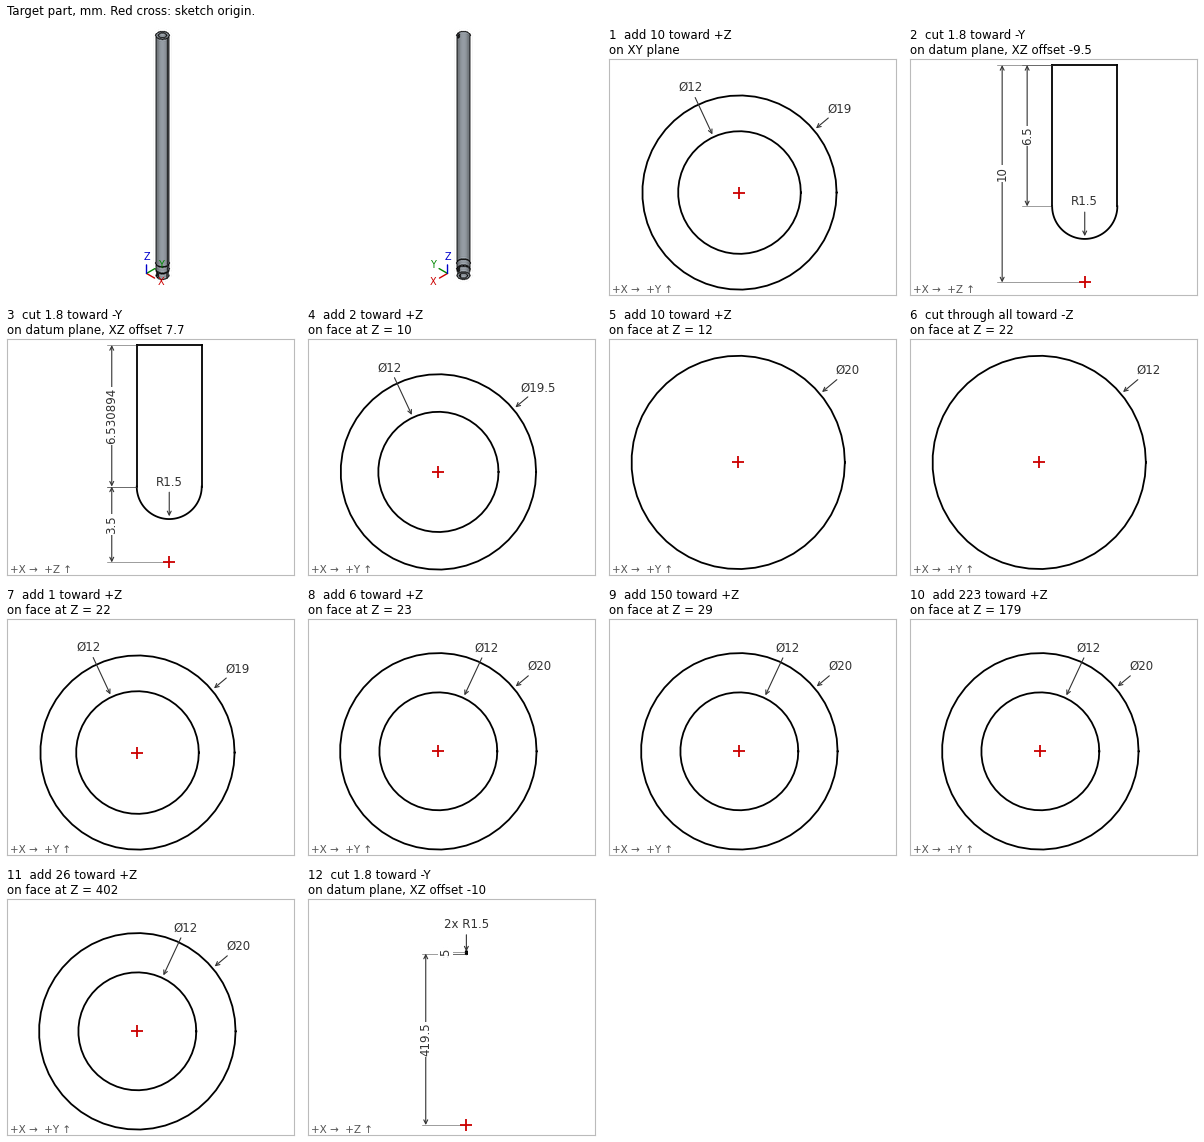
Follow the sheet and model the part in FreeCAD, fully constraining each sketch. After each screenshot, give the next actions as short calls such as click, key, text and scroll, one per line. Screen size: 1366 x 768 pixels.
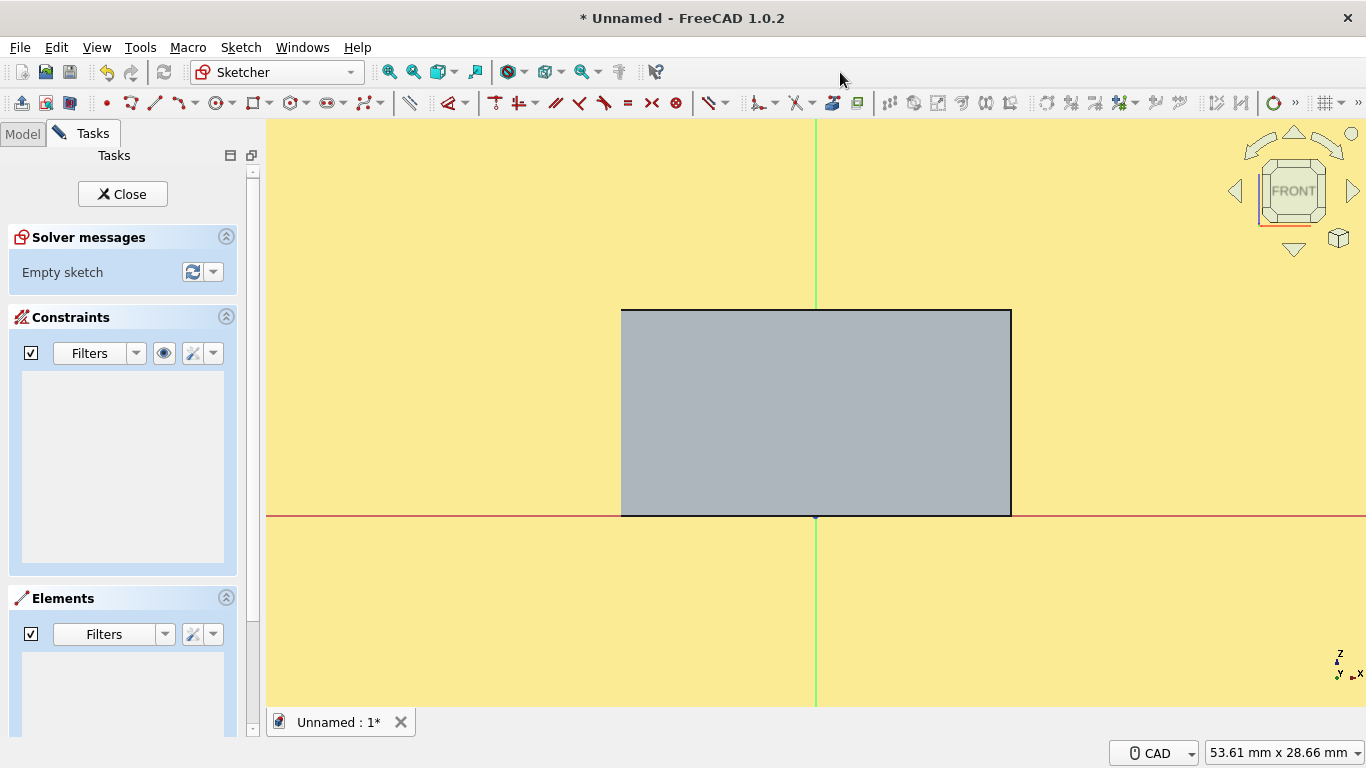
click(70, 104)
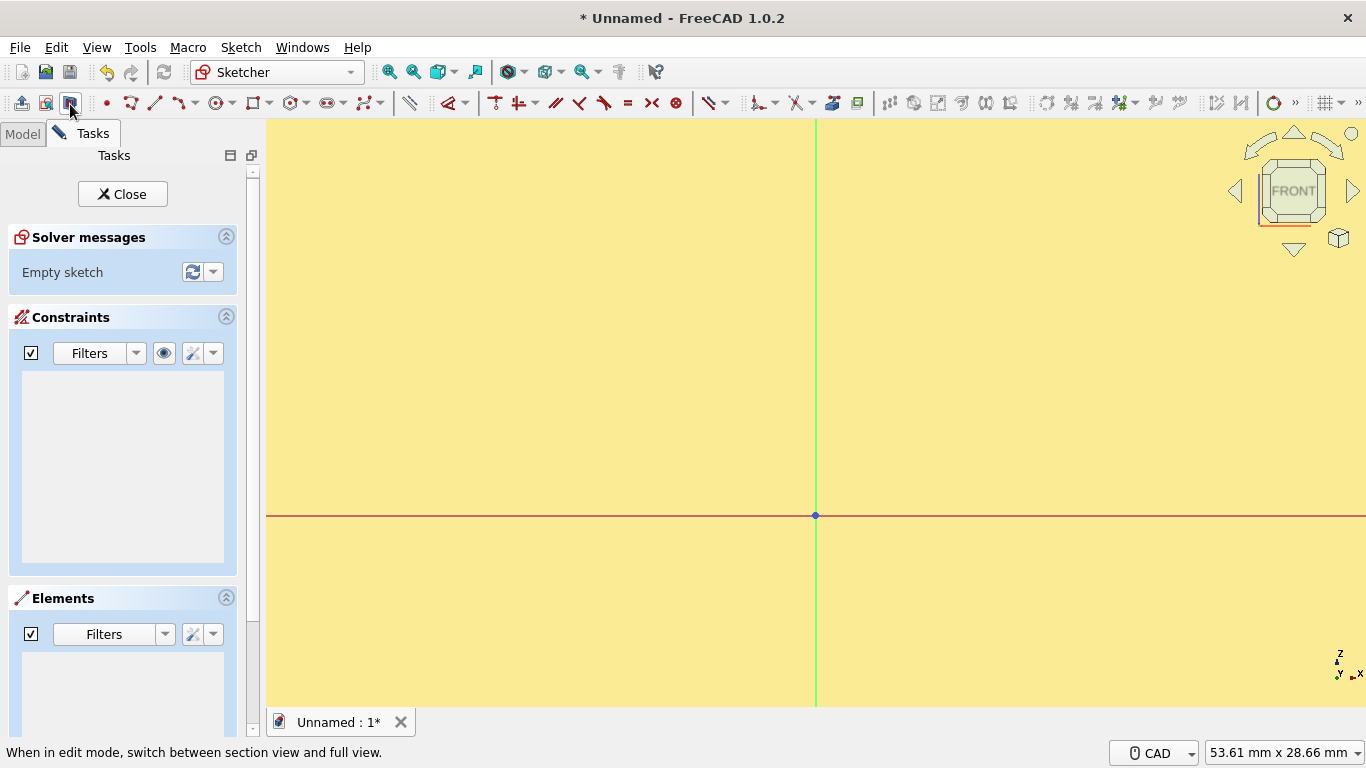
scroll(899, 413, up, 3)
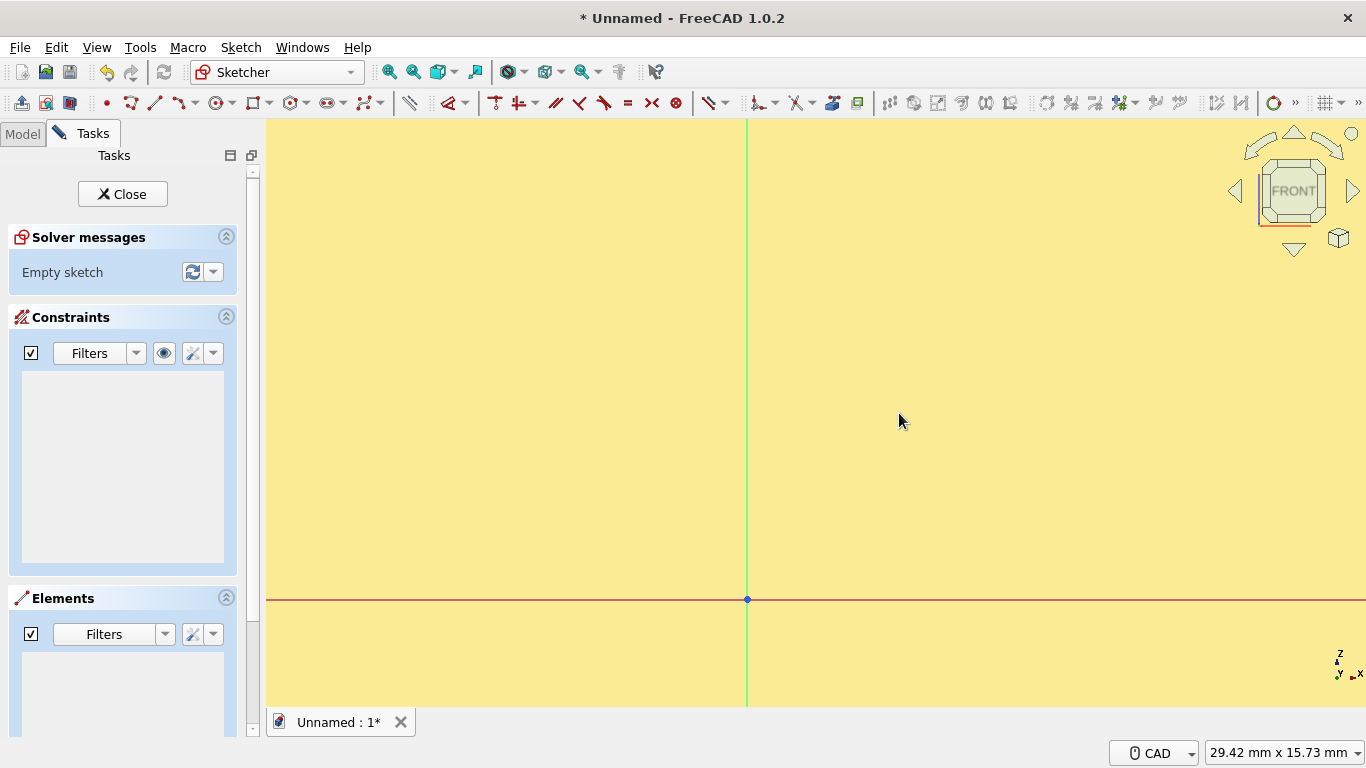
click(132, 104)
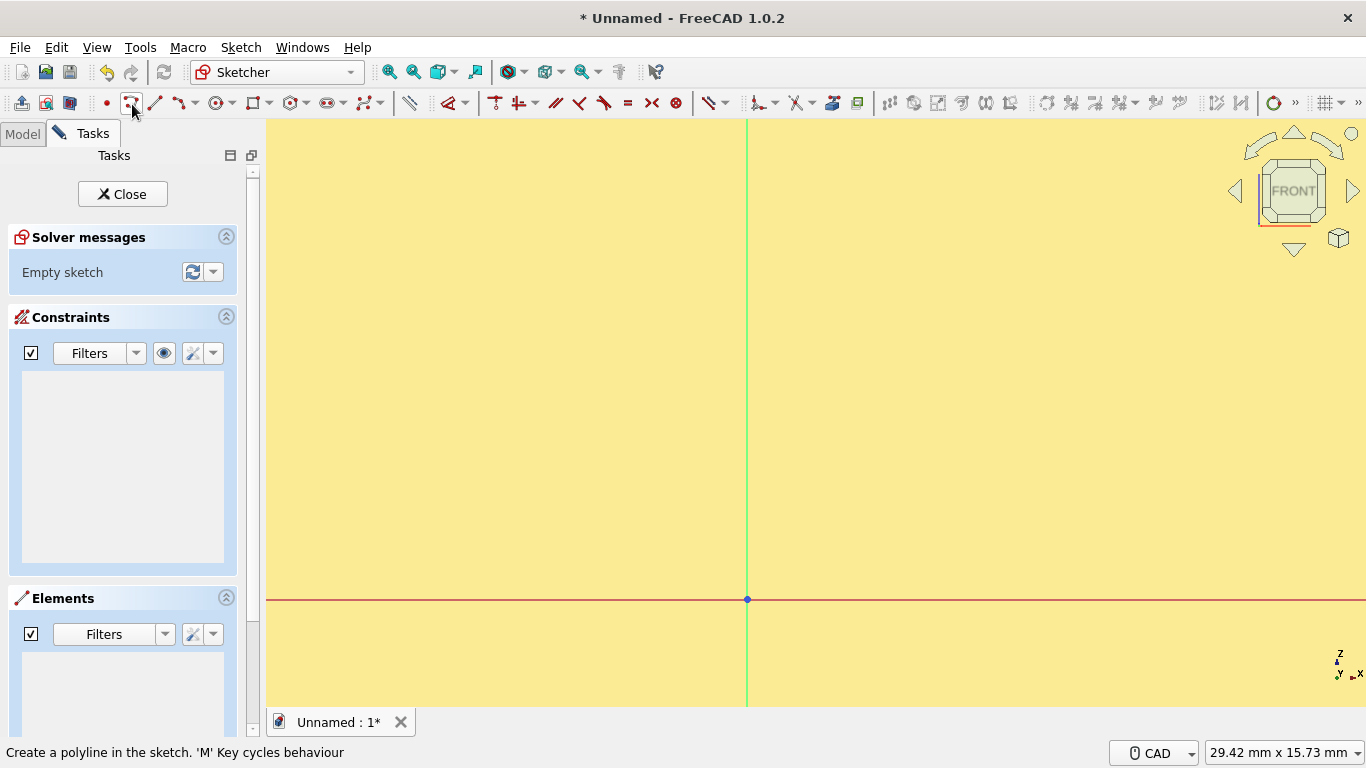
click(691, 469)
click(691, 226)
click(803, 226)
click(803, 469)
right_click(803, 469)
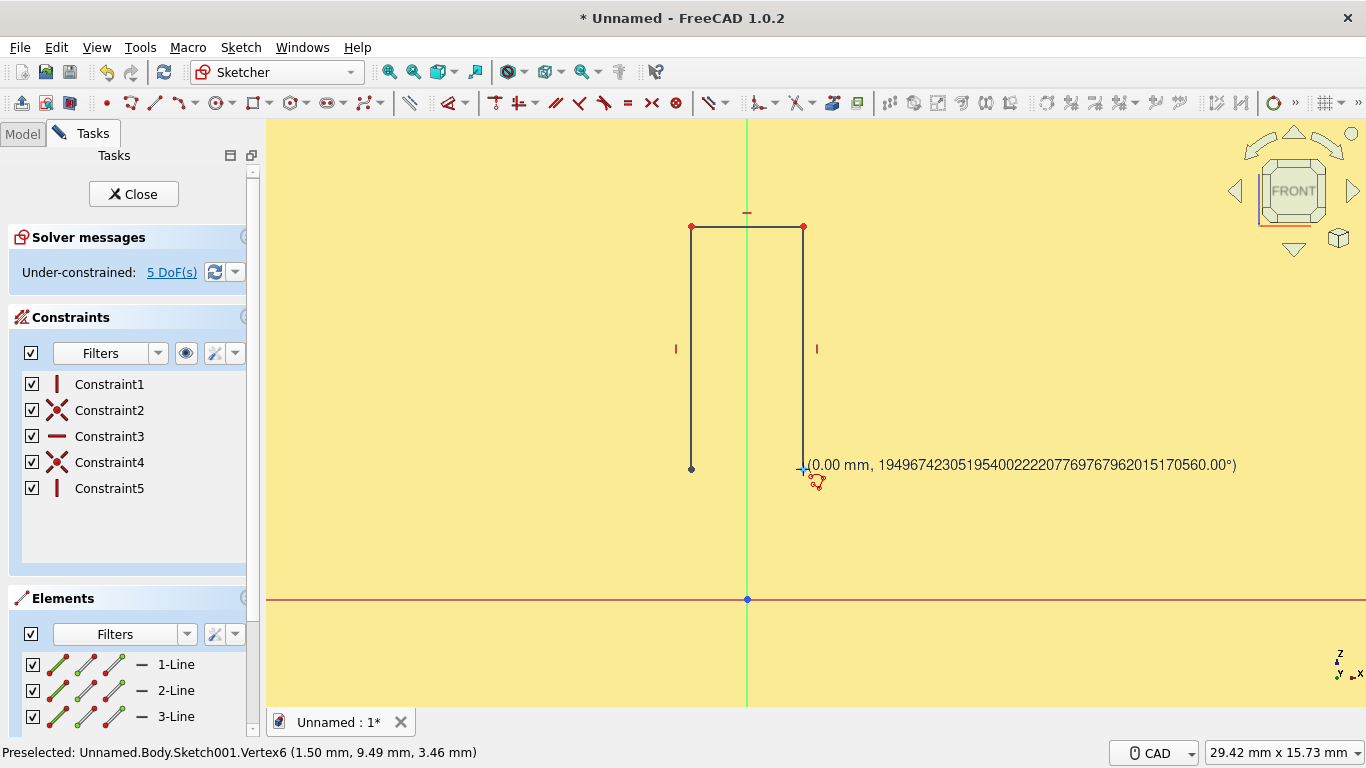
click(180, 104)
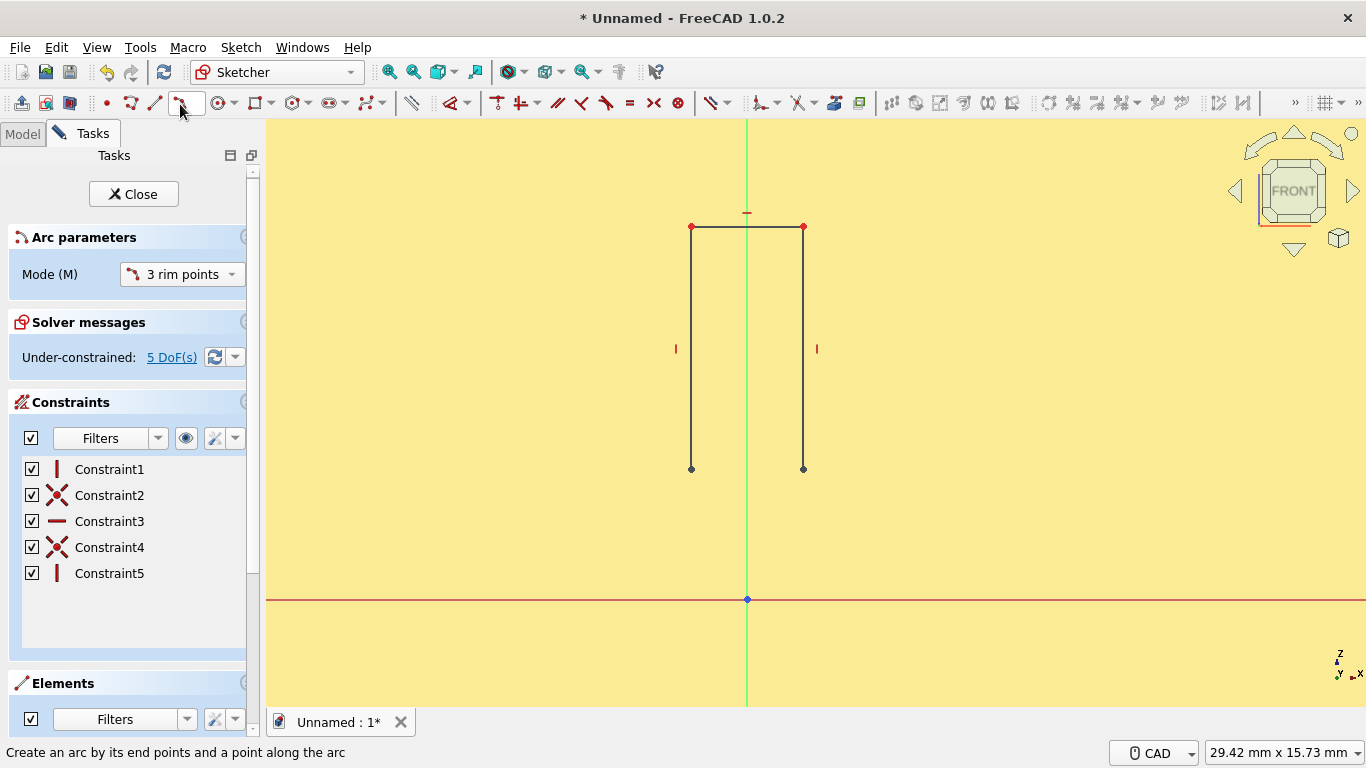
click(803, 470)
click(691, 470)
click(730, 522)
key(Escape)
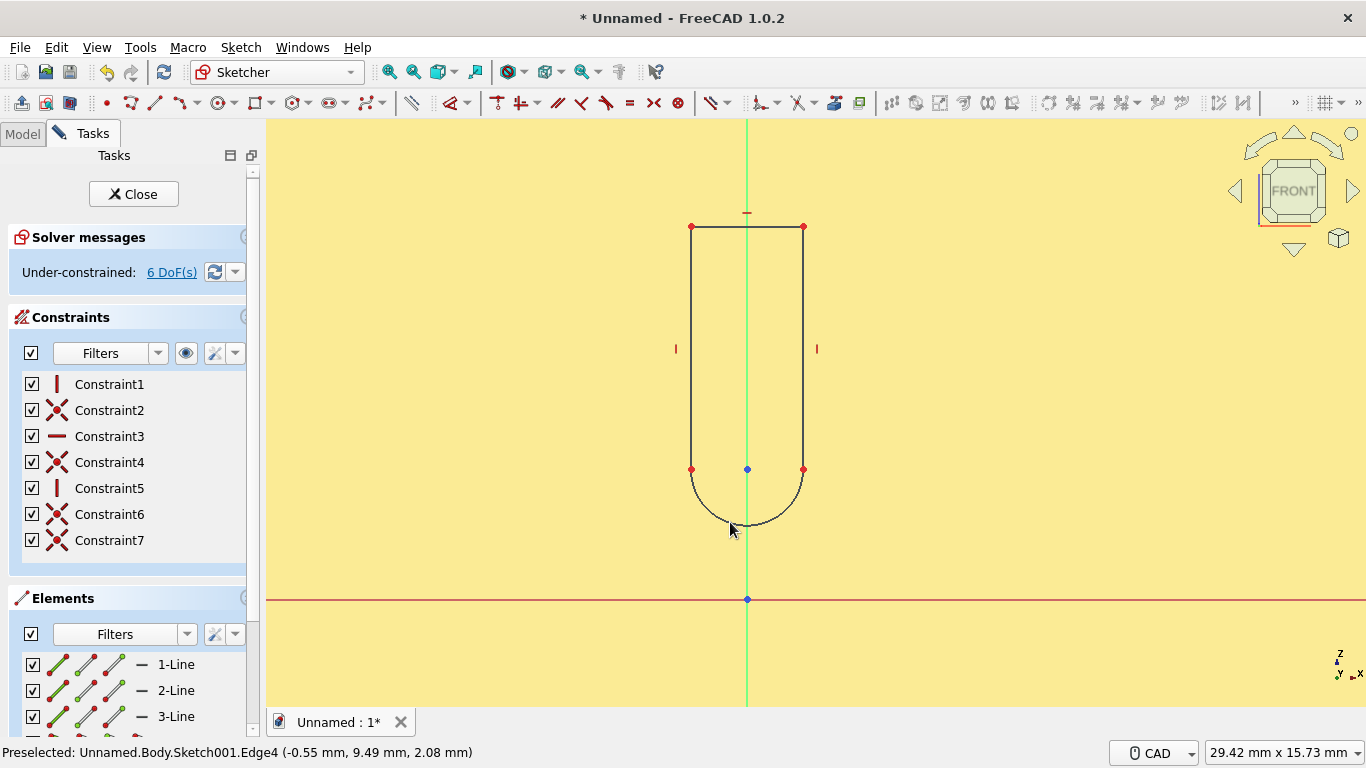
click(691, 397)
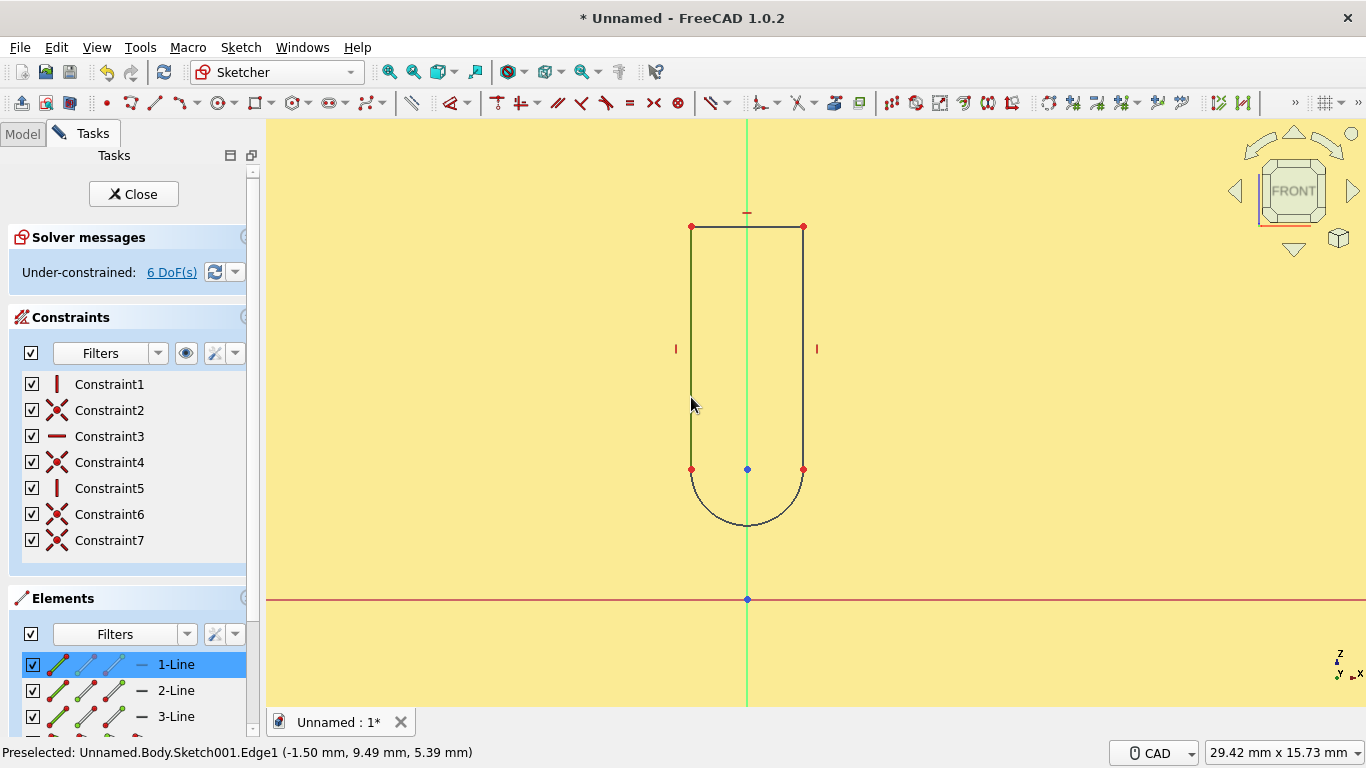
click(714, 515)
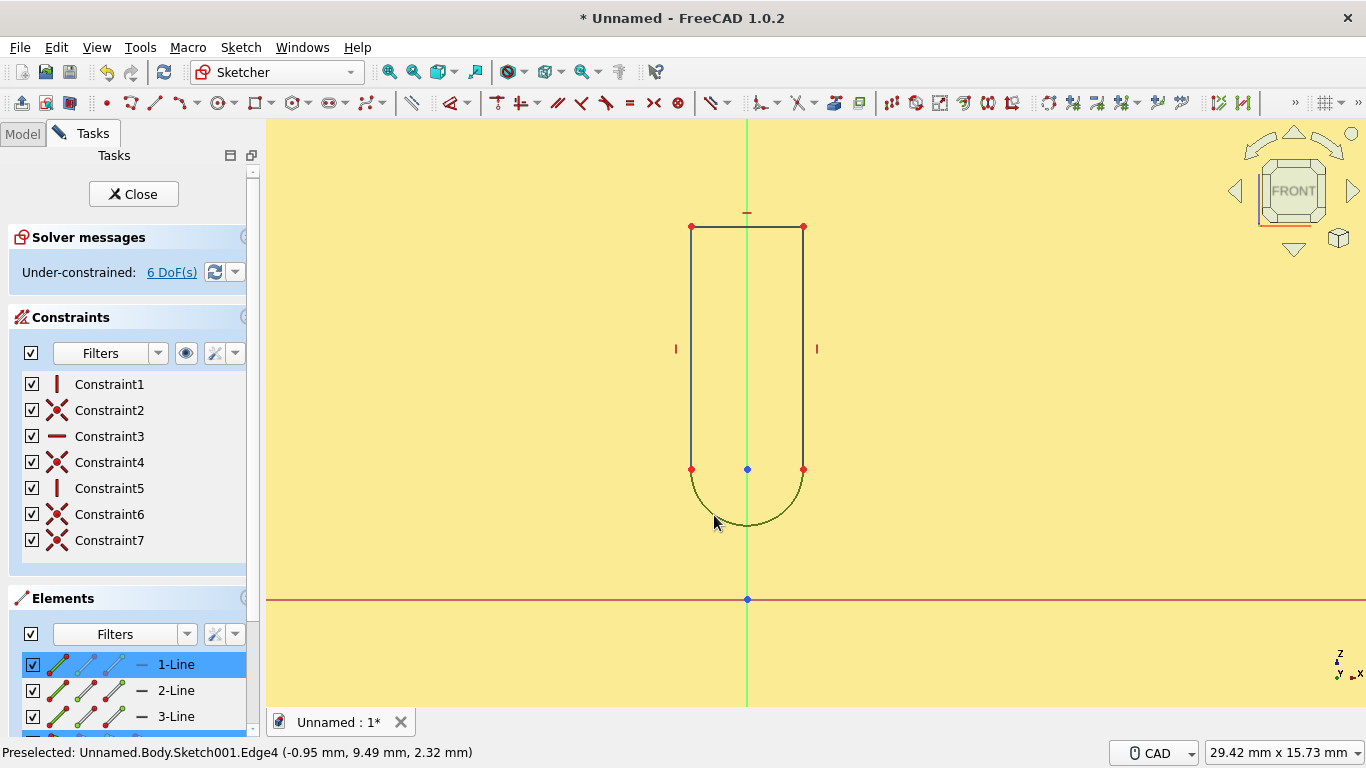
click(606, 104)